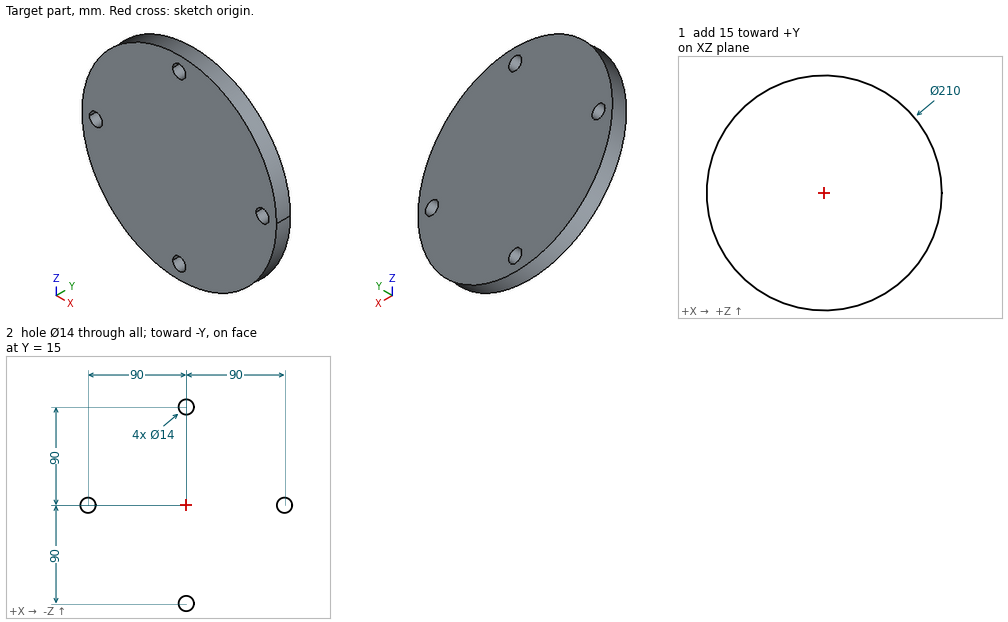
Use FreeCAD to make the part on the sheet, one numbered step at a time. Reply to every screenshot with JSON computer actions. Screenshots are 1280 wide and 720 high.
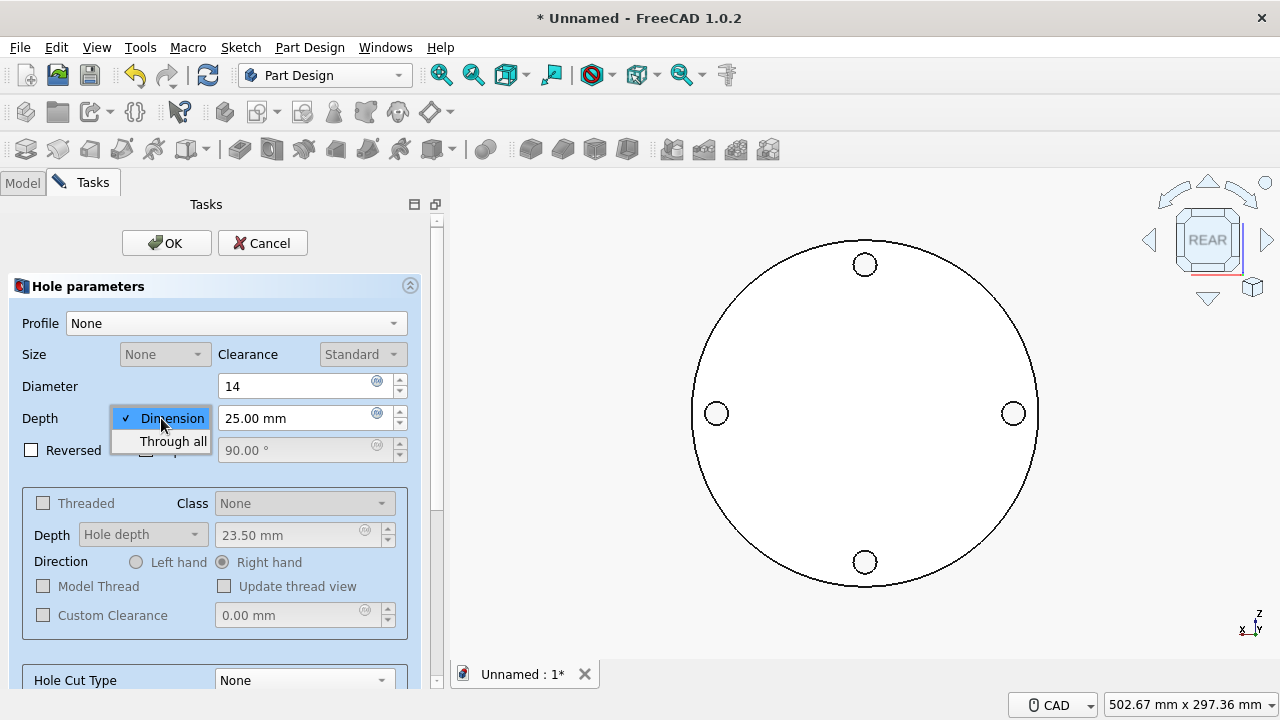
{"action": "left_click", "coordinate": [160, 442]}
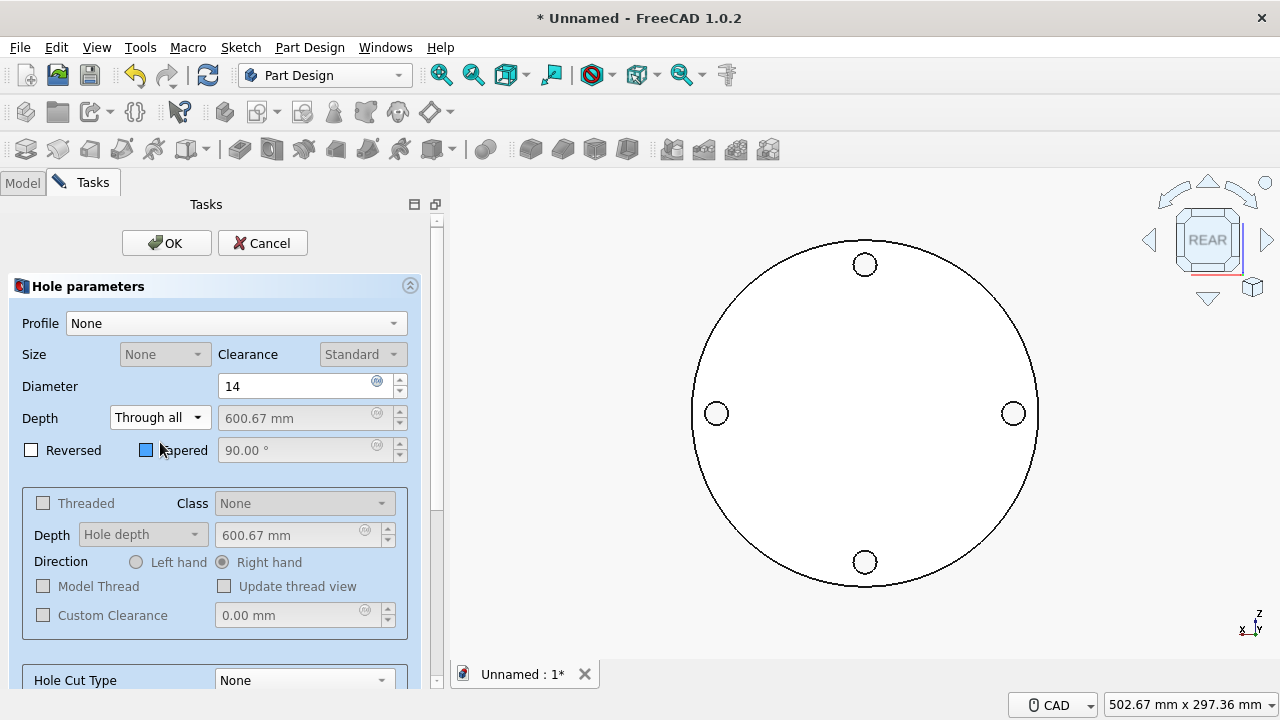
{"action": "left_click", "coordinate": [167, 243]}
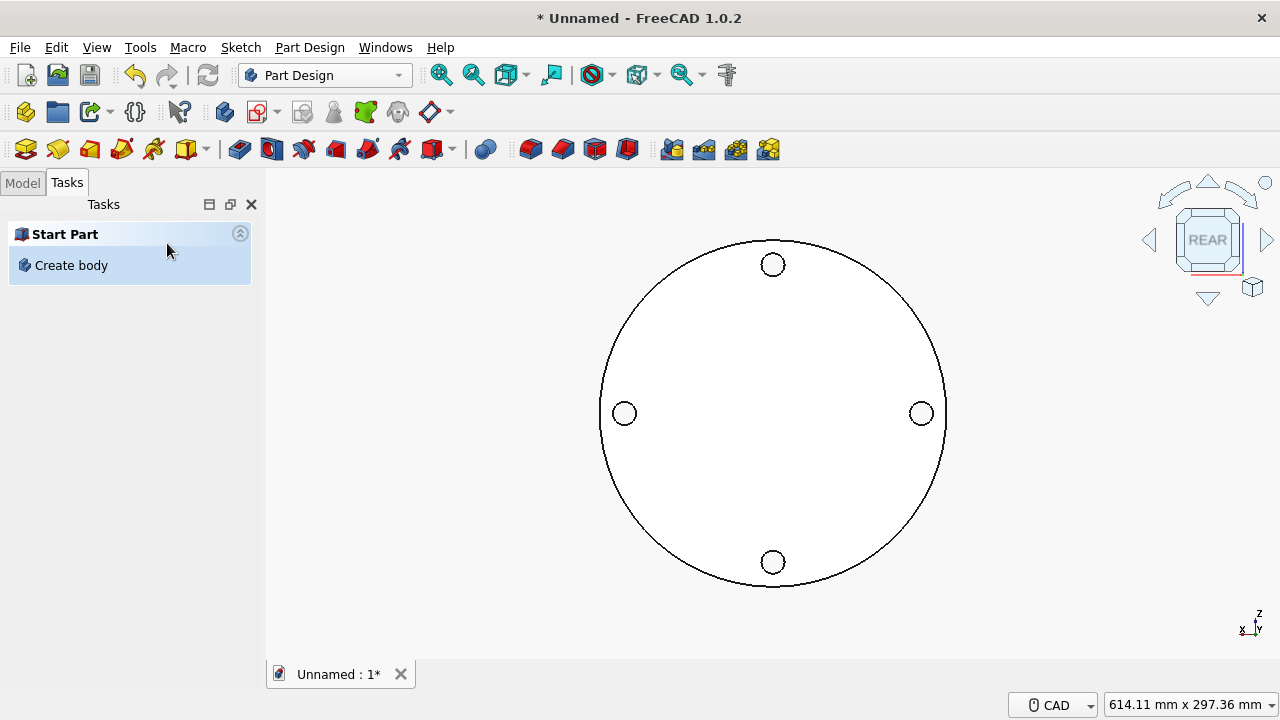
{"action": "key", "text": "0"}